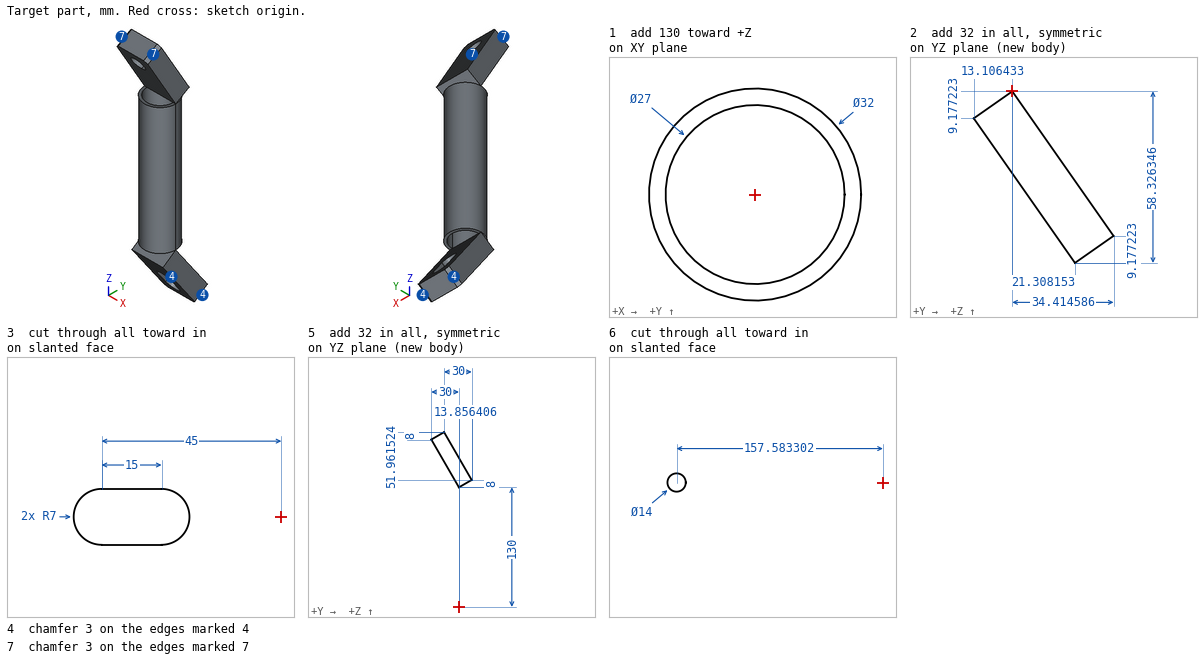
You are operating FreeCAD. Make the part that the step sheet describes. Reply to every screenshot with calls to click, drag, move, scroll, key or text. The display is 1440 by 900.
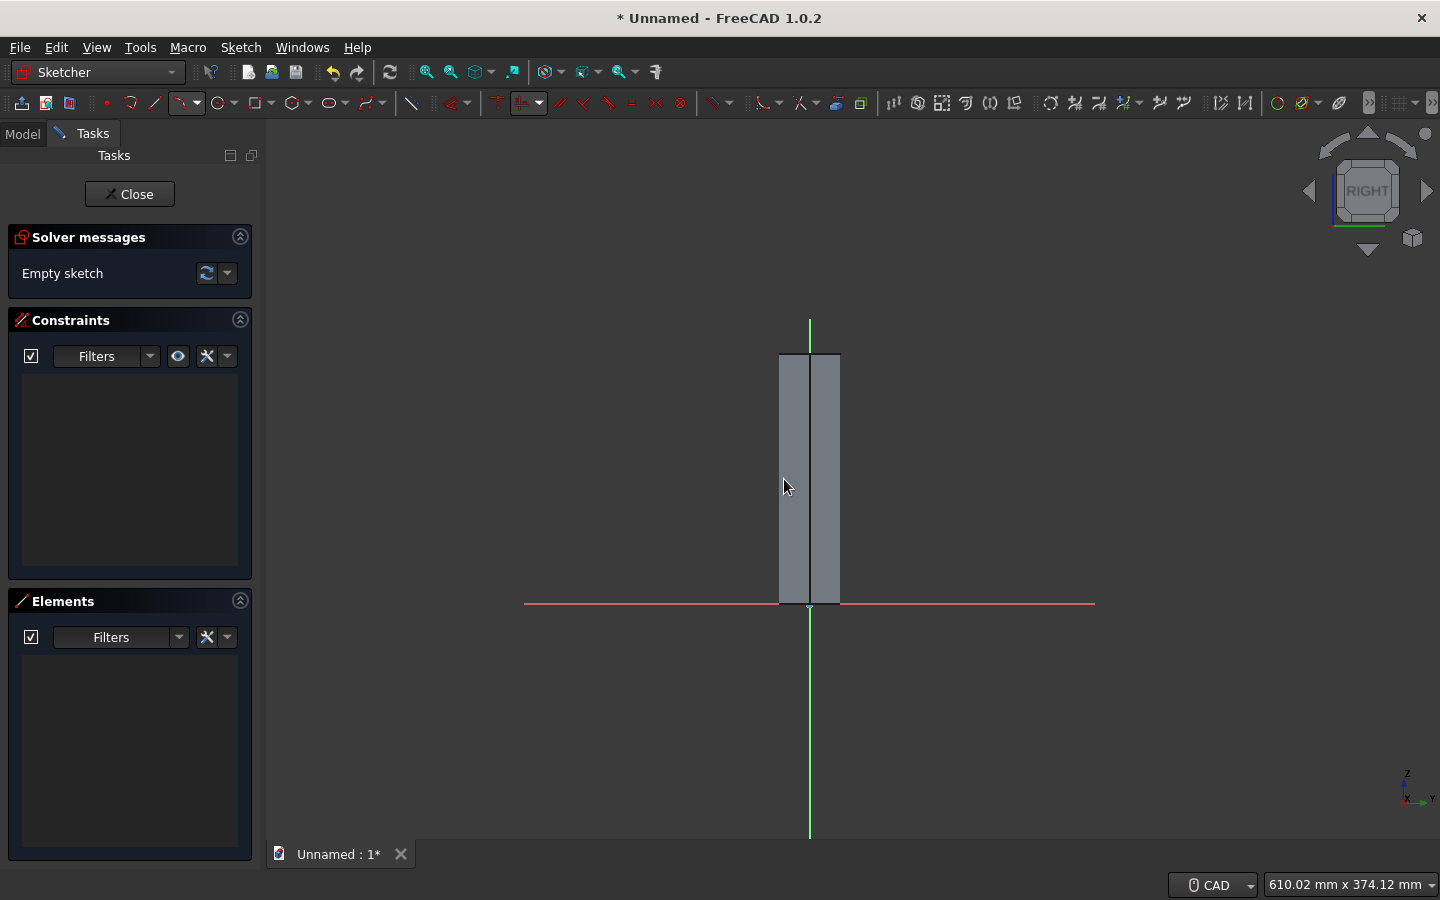
scroll(845, 720, up, 7)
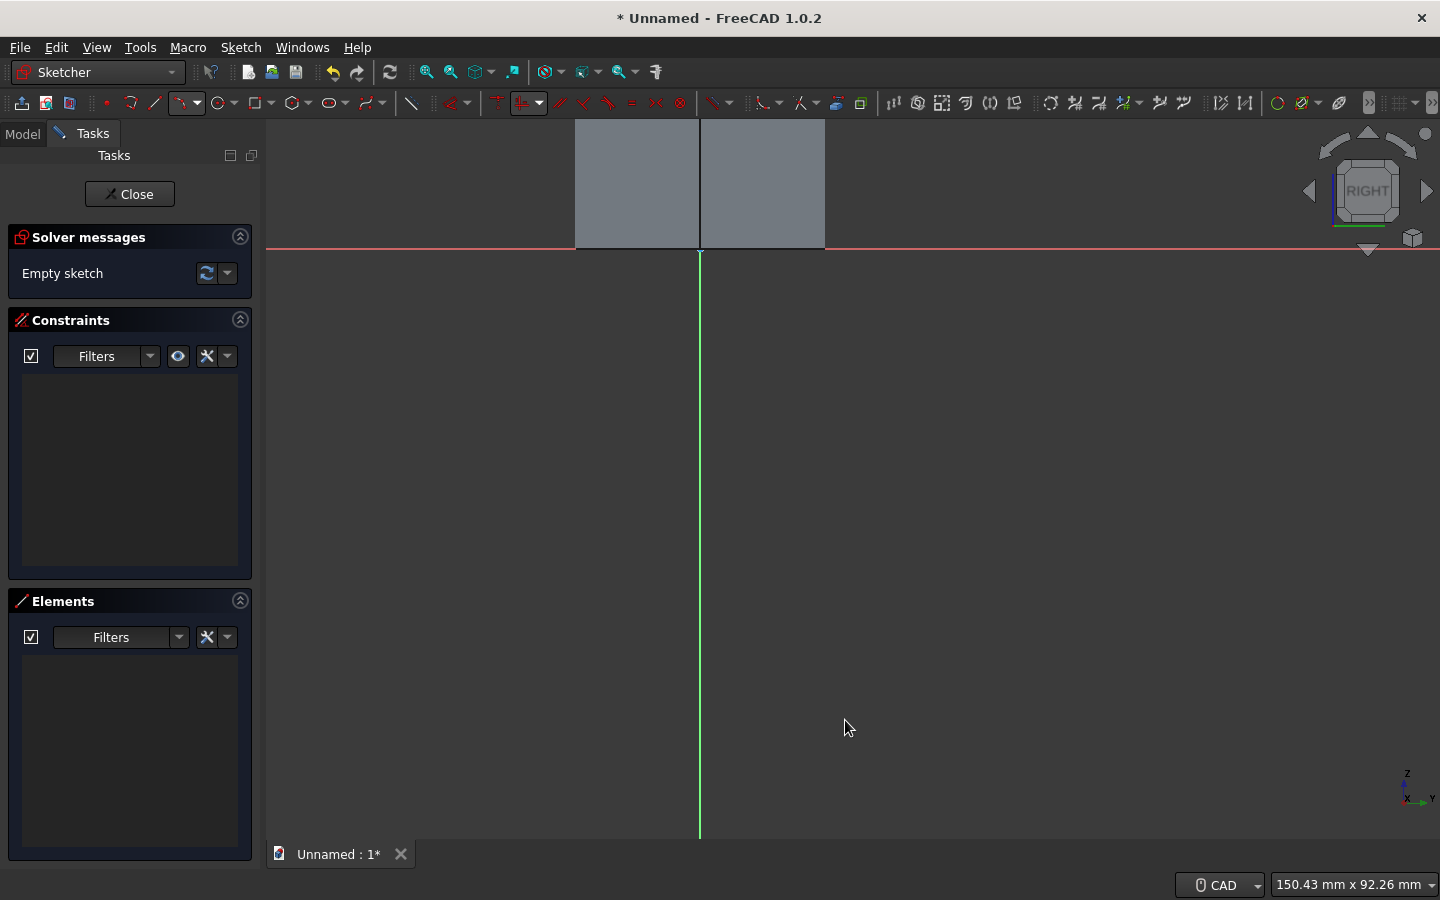
key(g)
key(m)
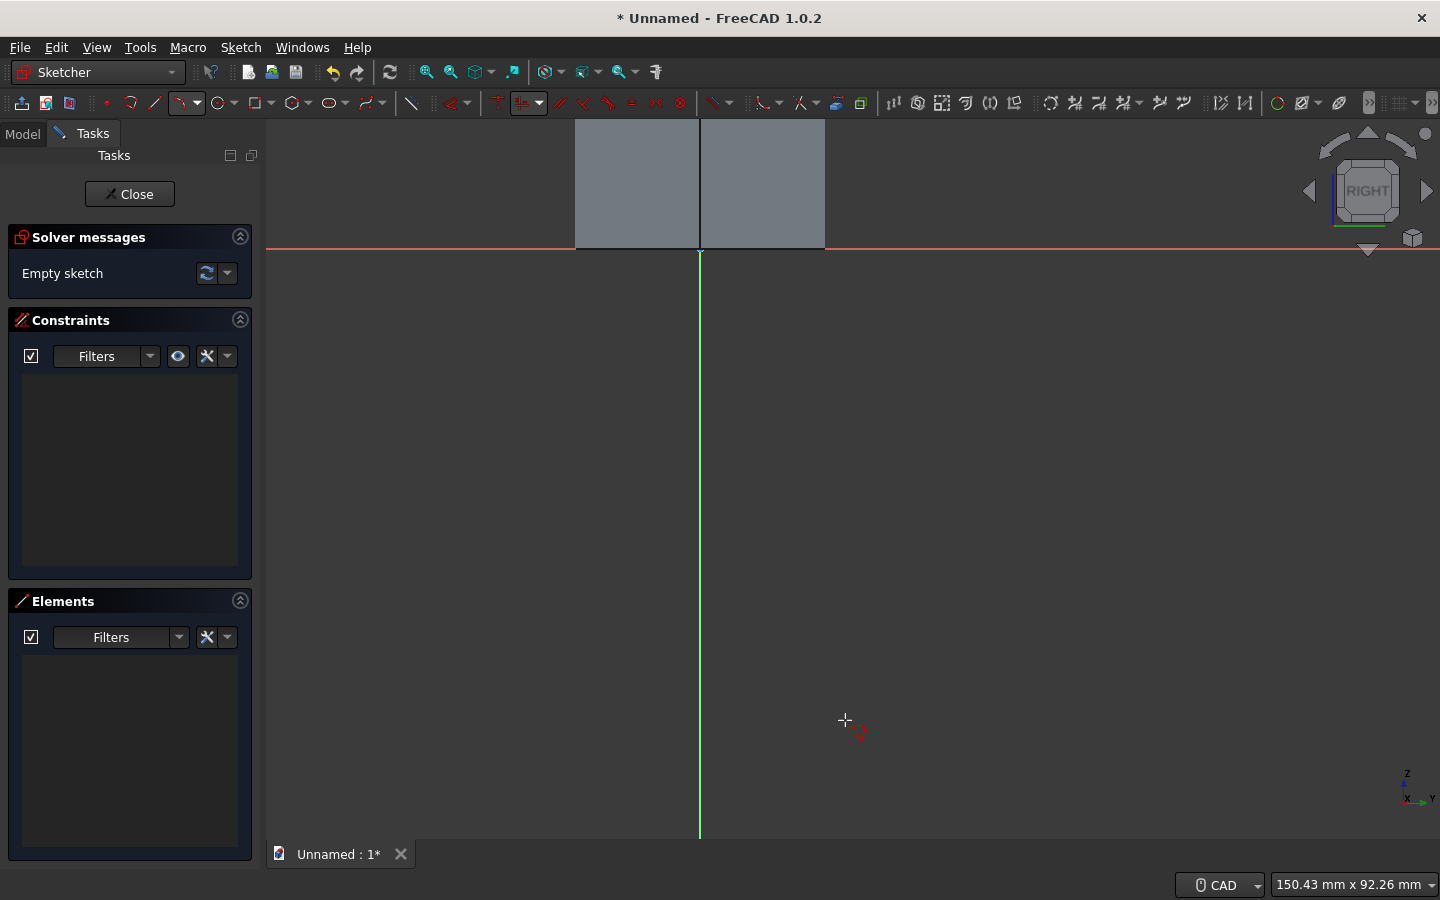
click(700, 249)
click(598, 320)
click(866, 704)
click(969, 632)
click(700, 249)
key(Escape)
key(Escape)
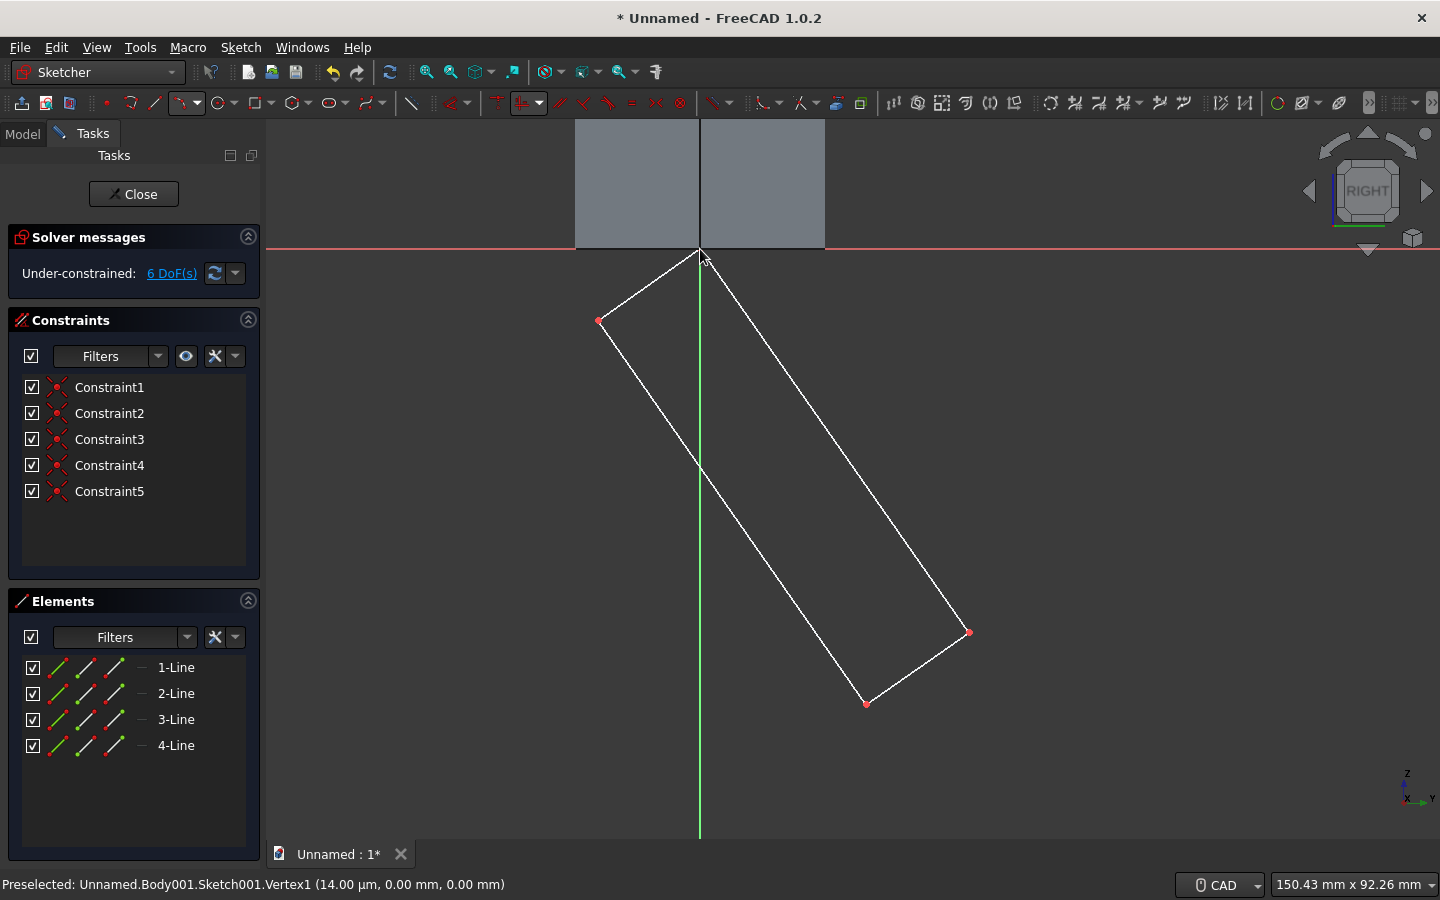
click(450, 104)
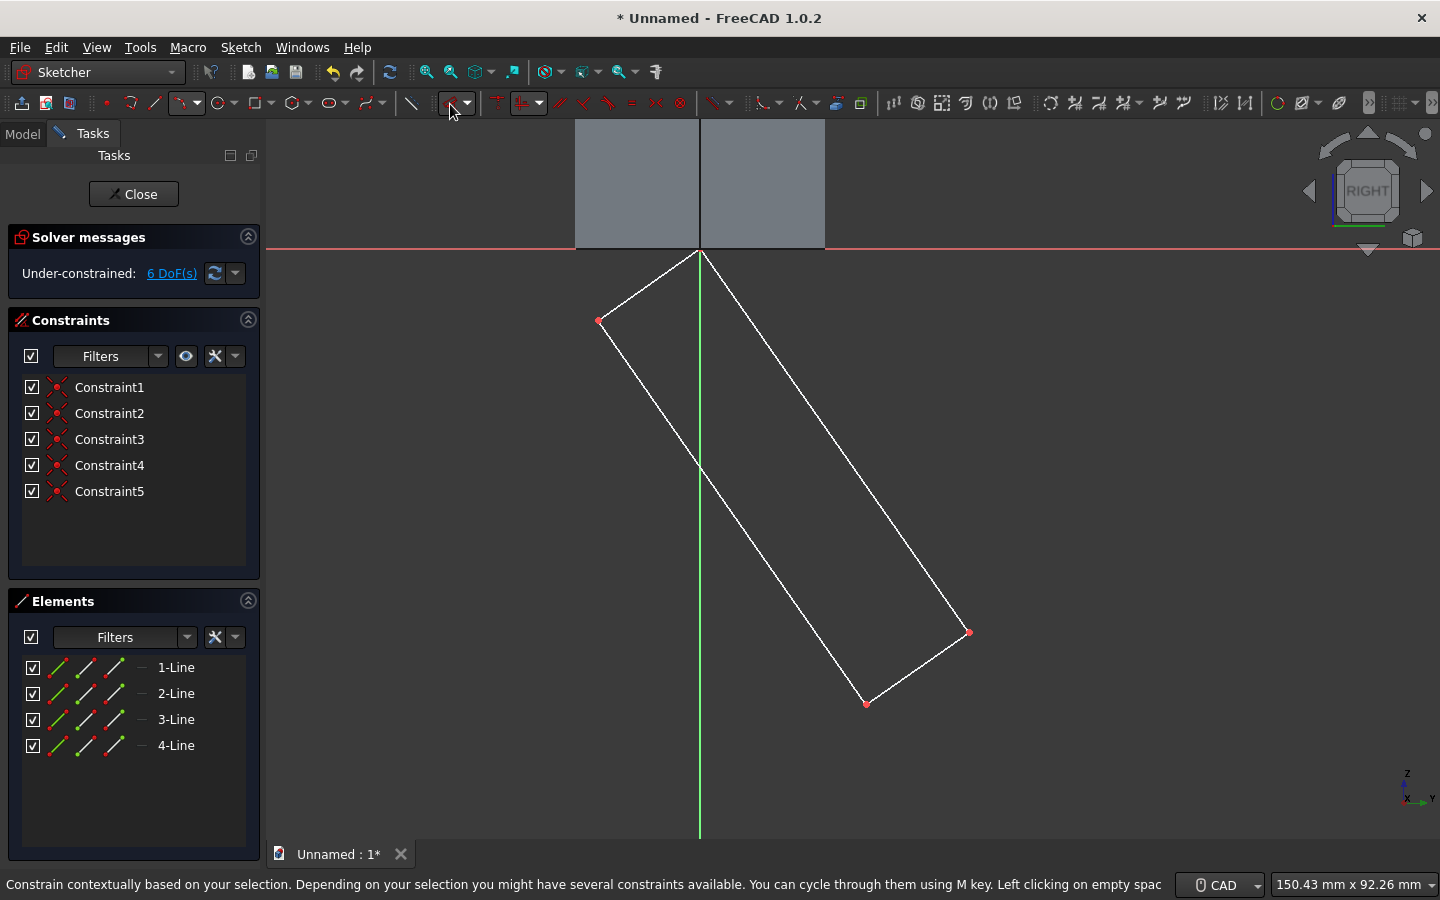
click(598, 321)
click(564, 285)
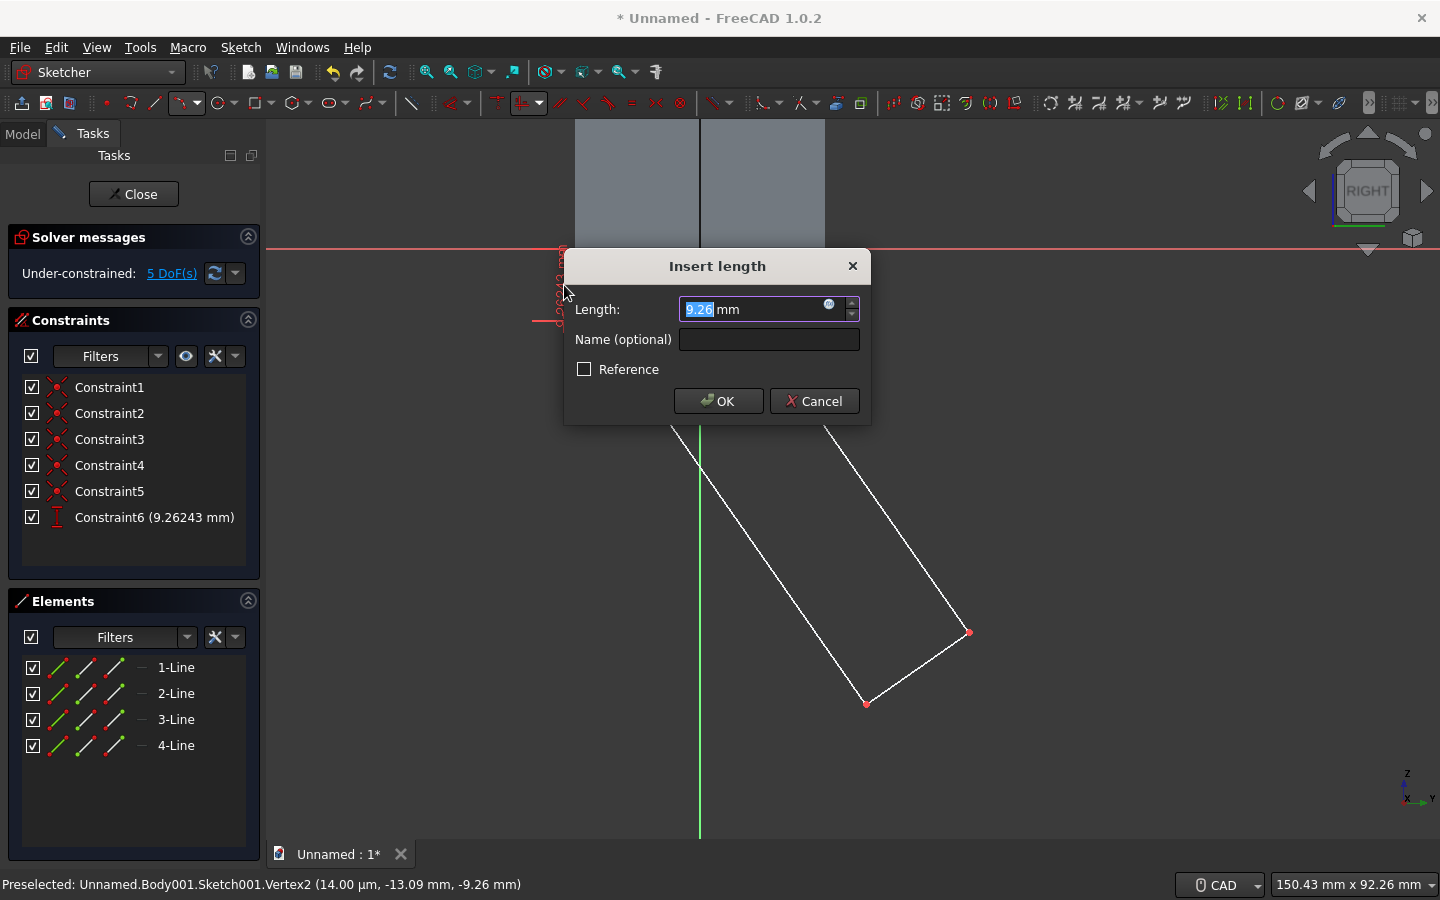
text(9.177223)
key(Return)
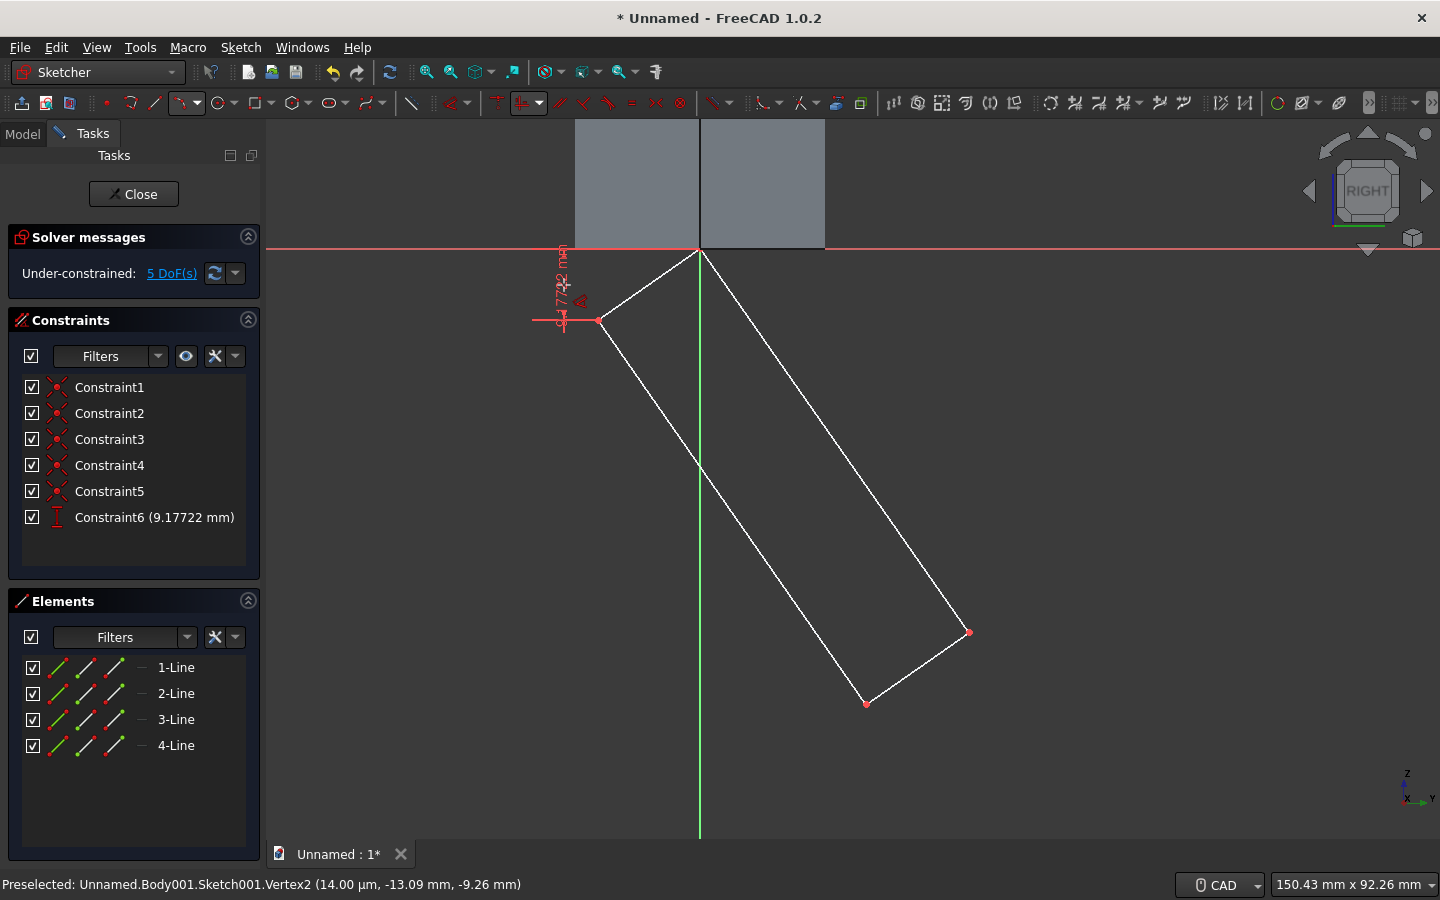
click(897, 683)
click(1003, 669)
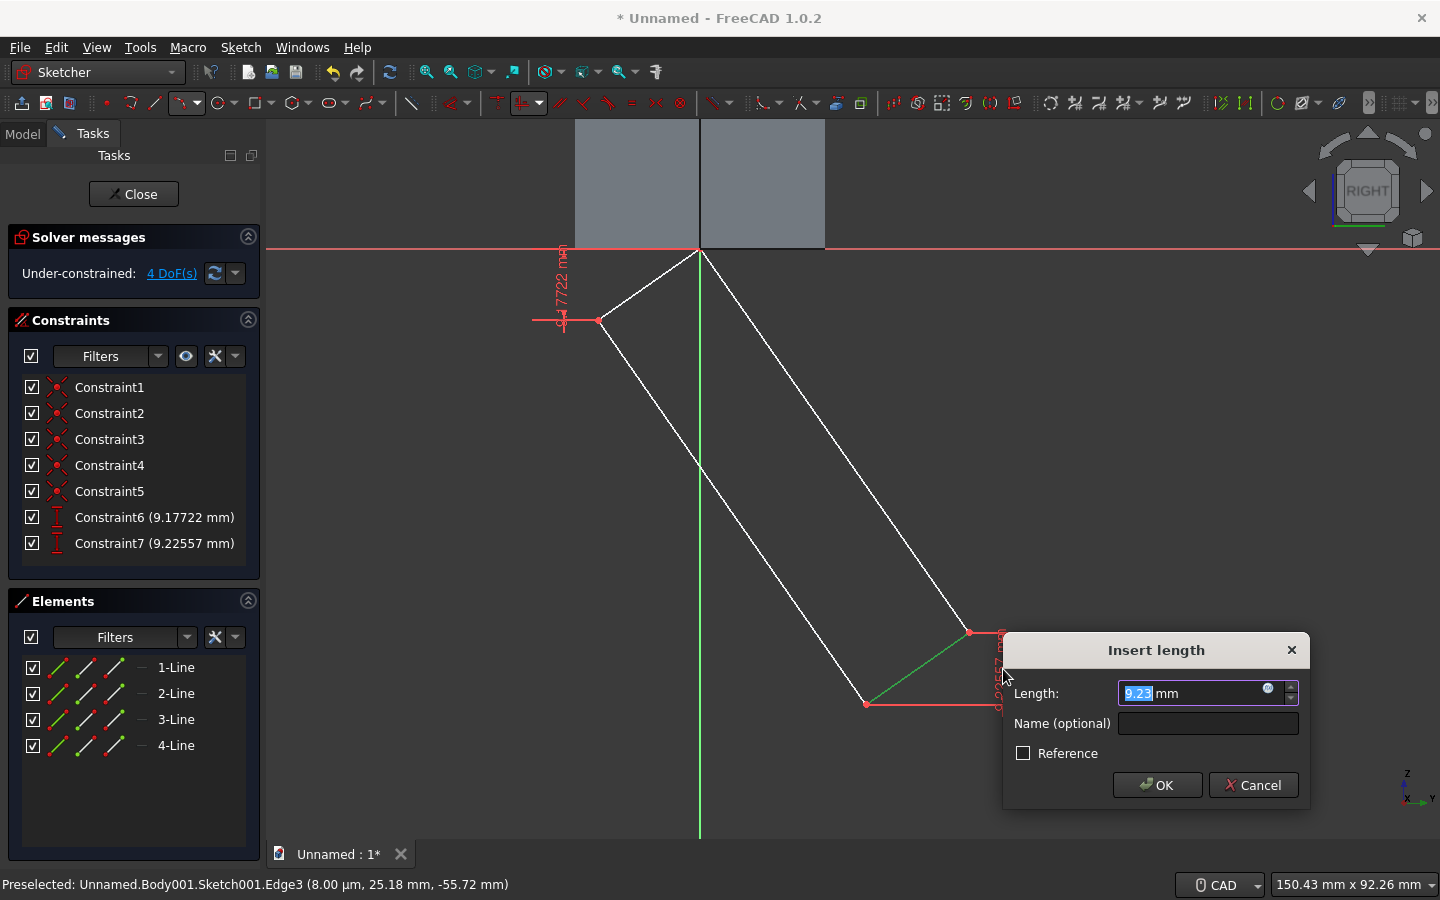
text(9.177223)
key(Return)